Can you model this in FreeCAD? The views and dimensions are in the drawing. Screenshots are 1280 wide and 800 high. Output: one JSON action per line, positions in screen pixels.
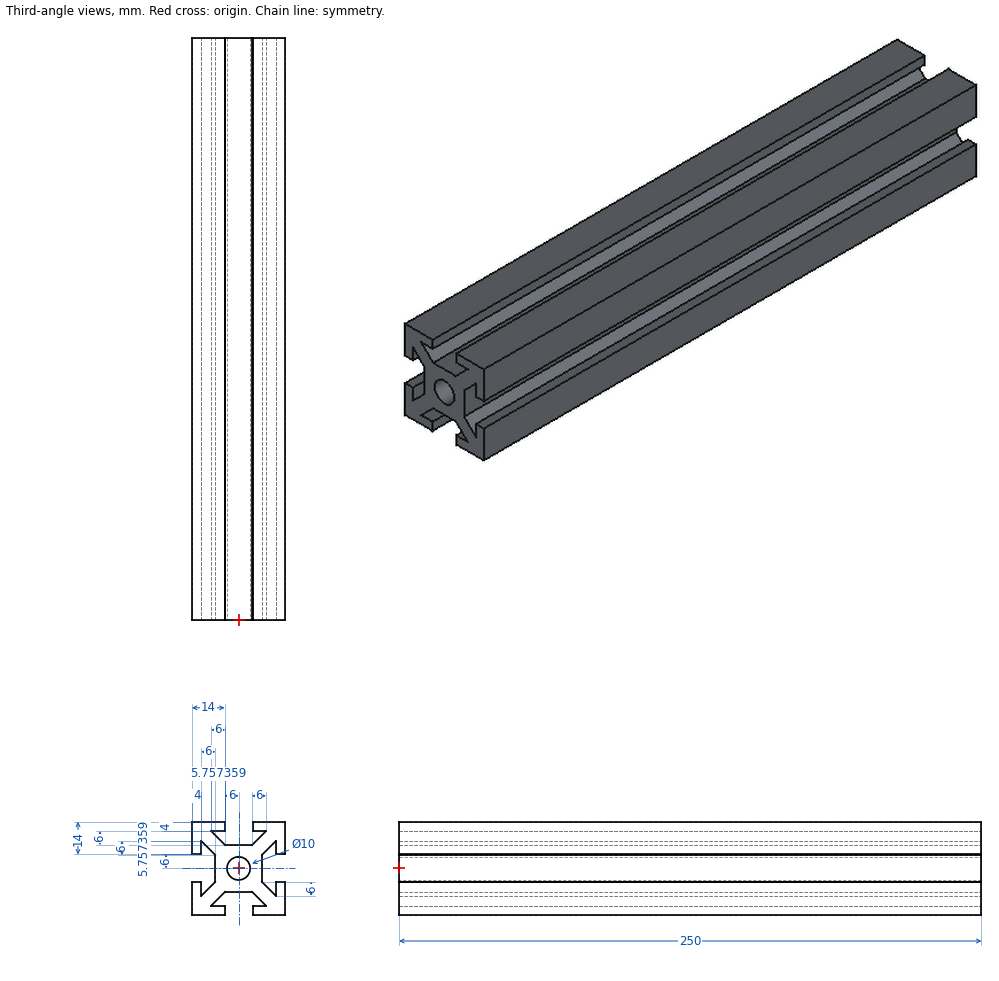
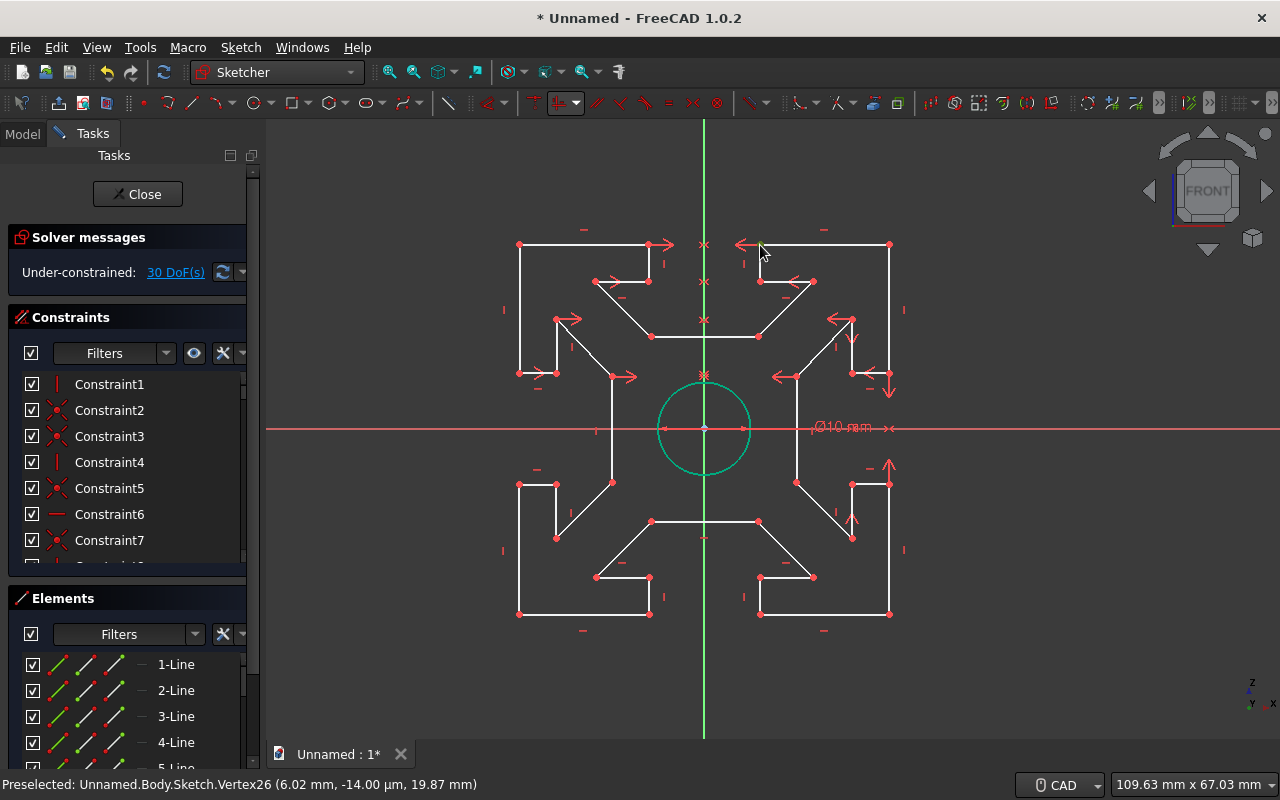
{"action": "left_click", "coordinate": [760, 615]}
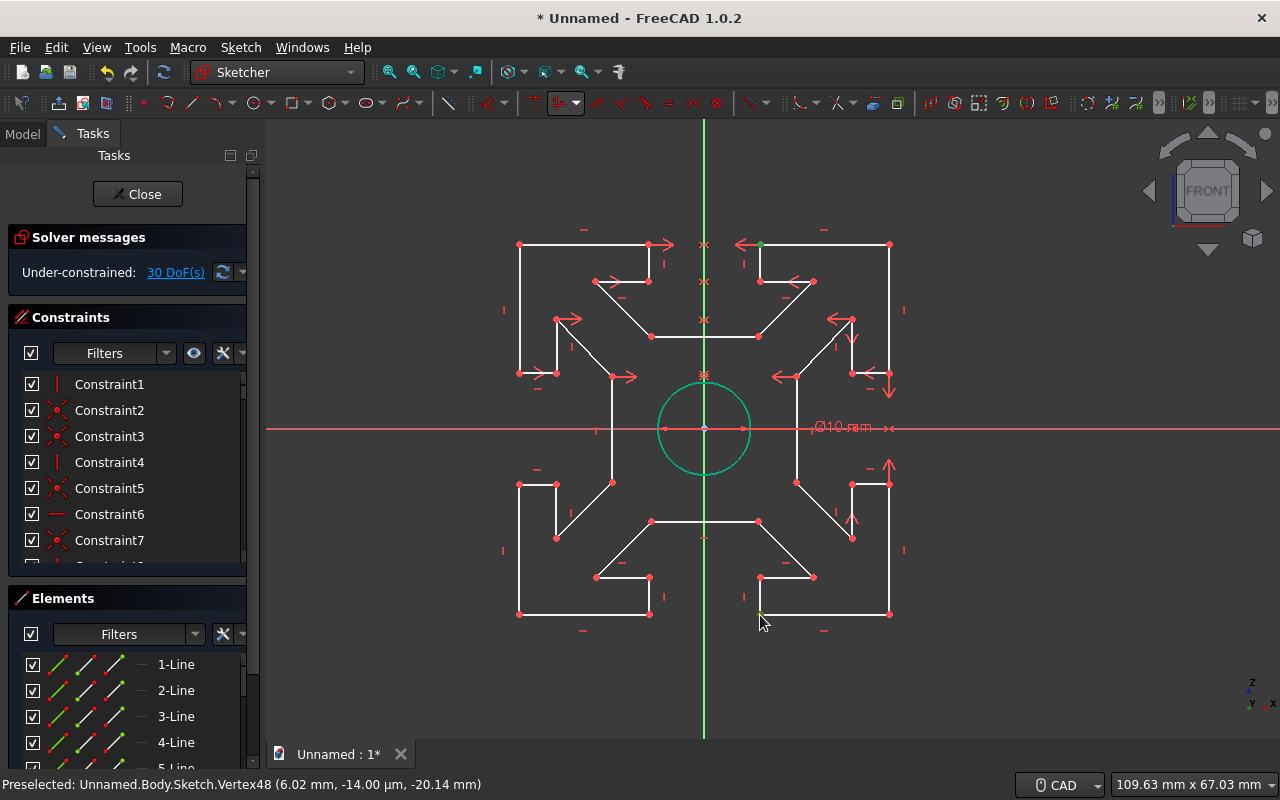
{"action": "left_click", "coordinate": [353, 429]}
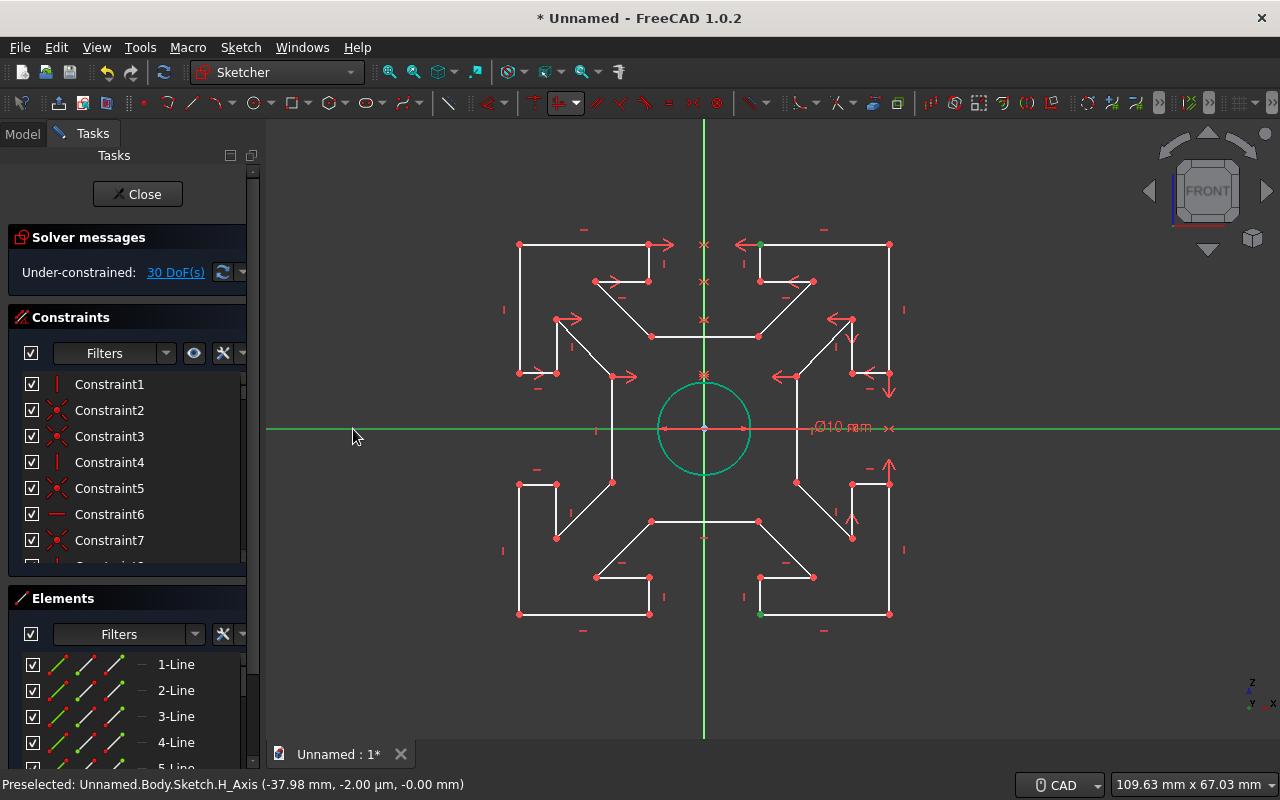
{"action": "left_click", "coordinate": [694, 104]}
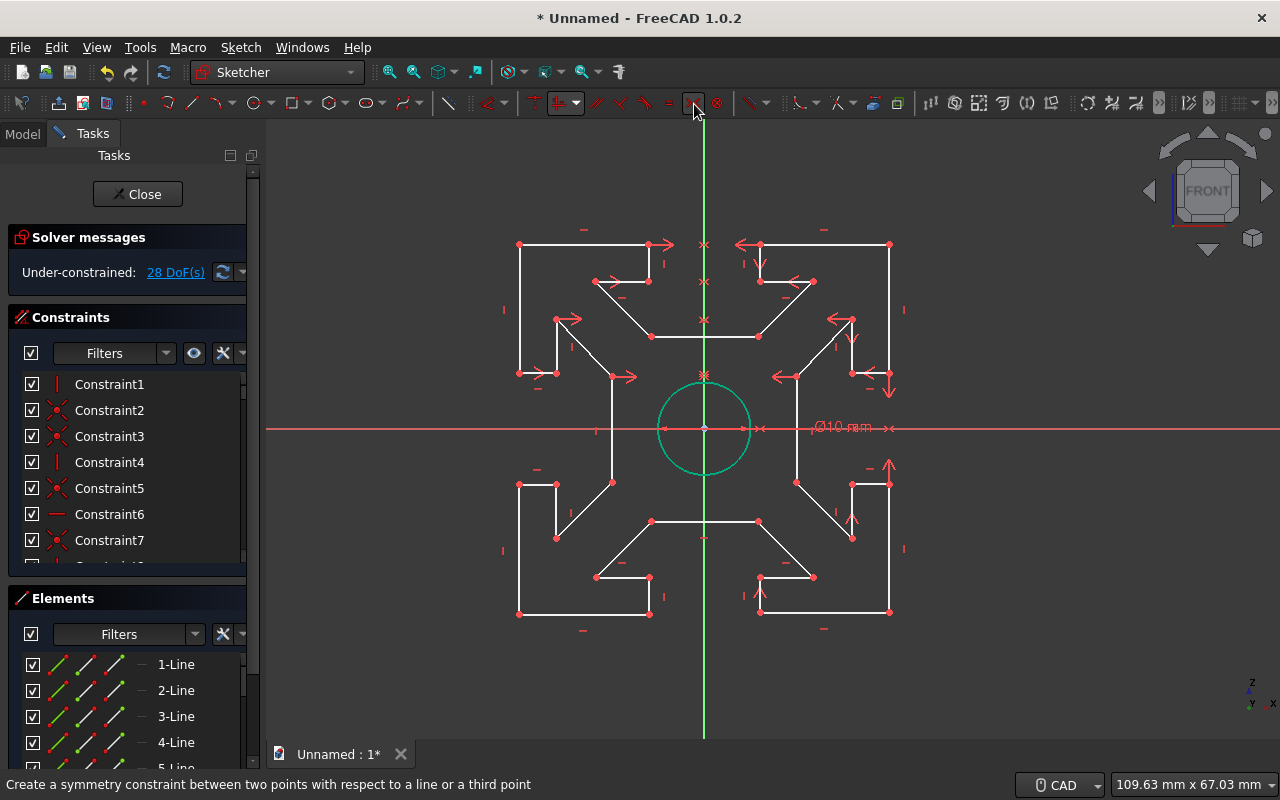
{"action": "left_click", "coordinate": [813, 282]}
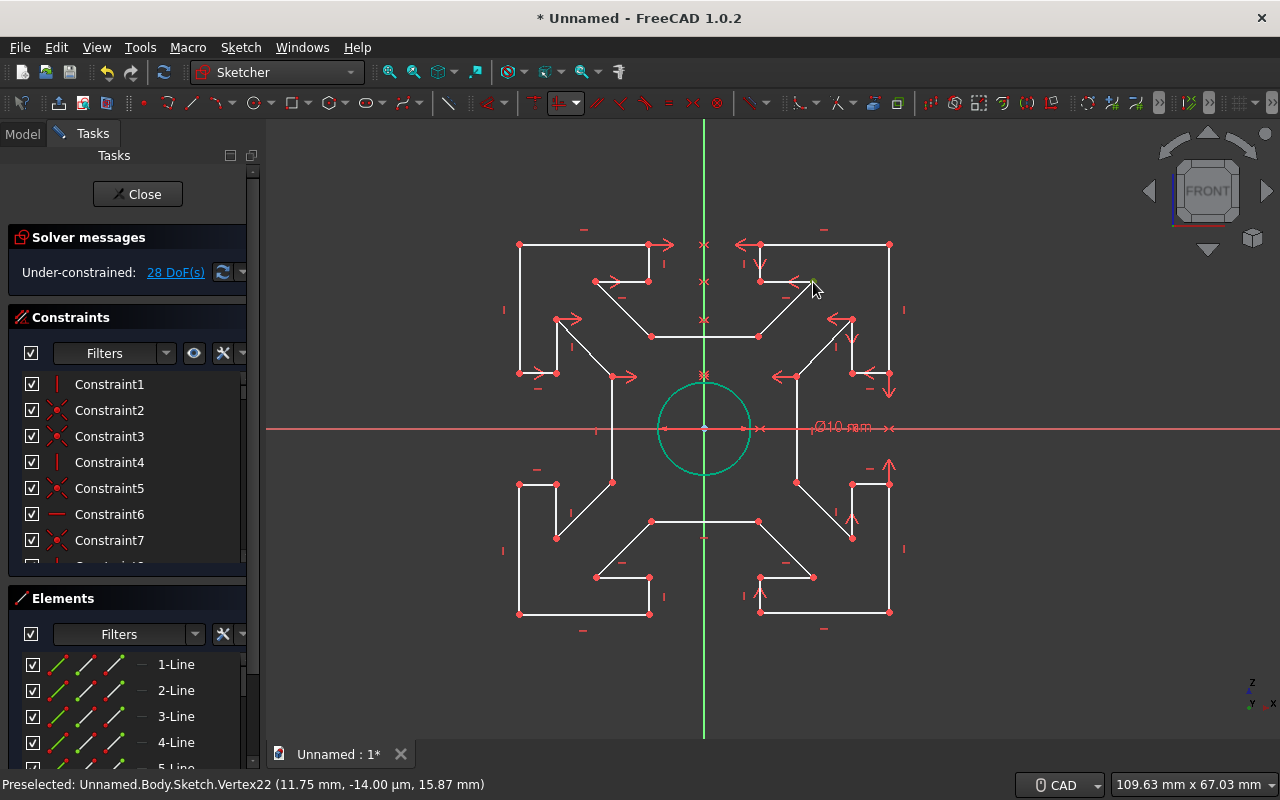
{"action": "left_click", "coordinate": [813, 578]}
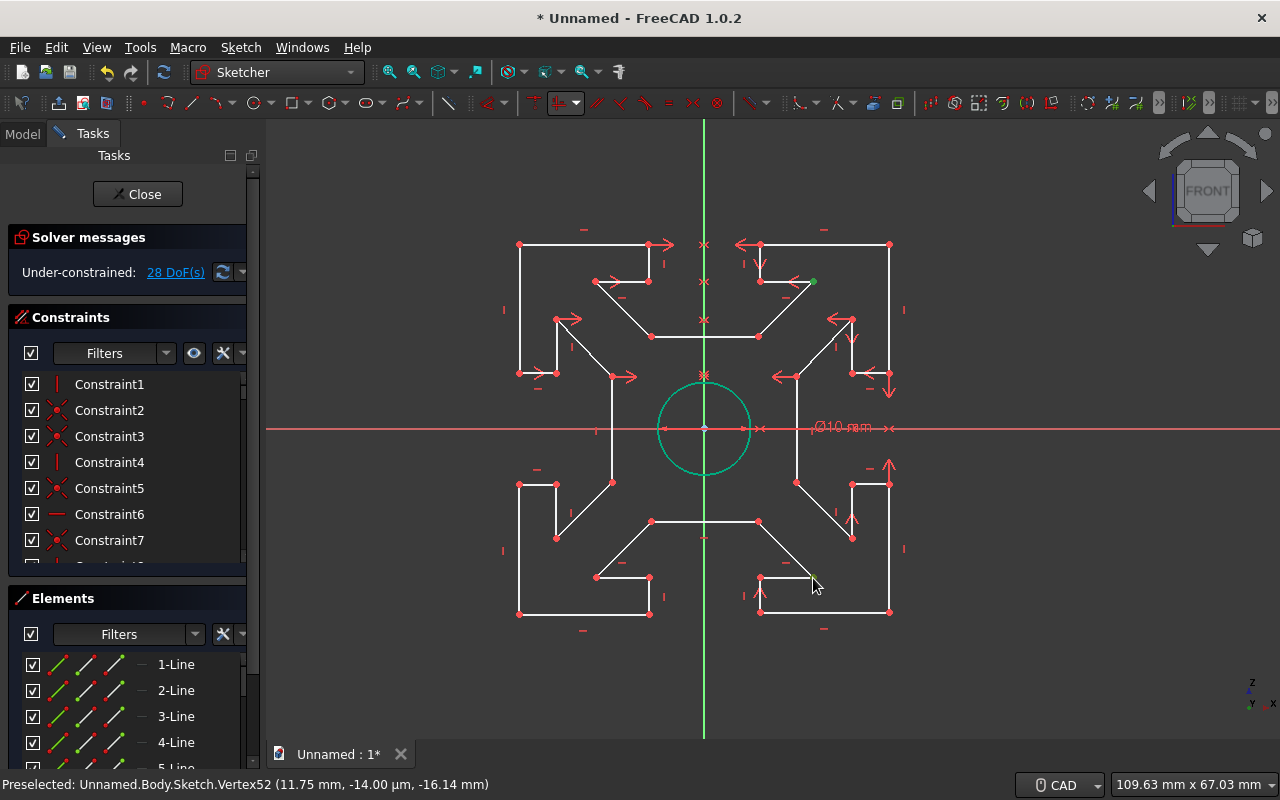
{"action": "left_click", "coordinate": [353, 429]}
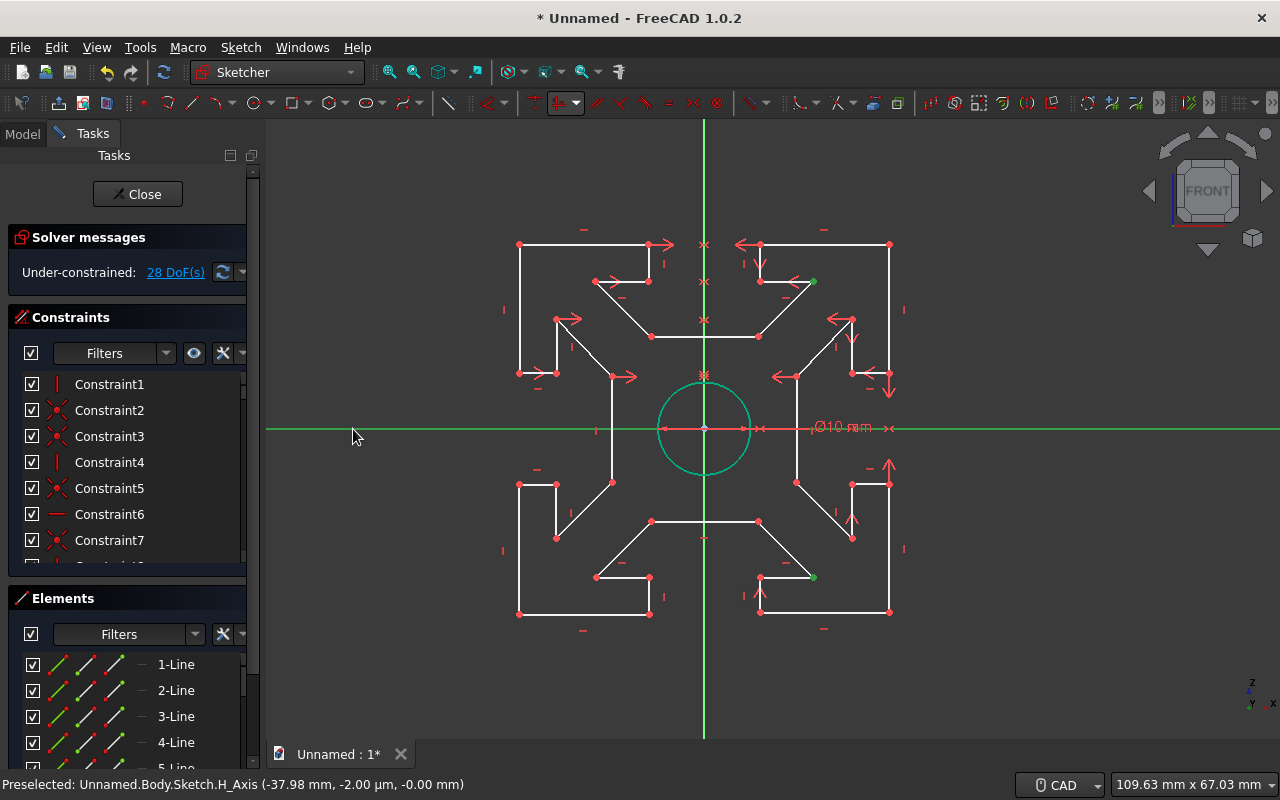
{"action": "left_click", "coordinate": [694, 104]}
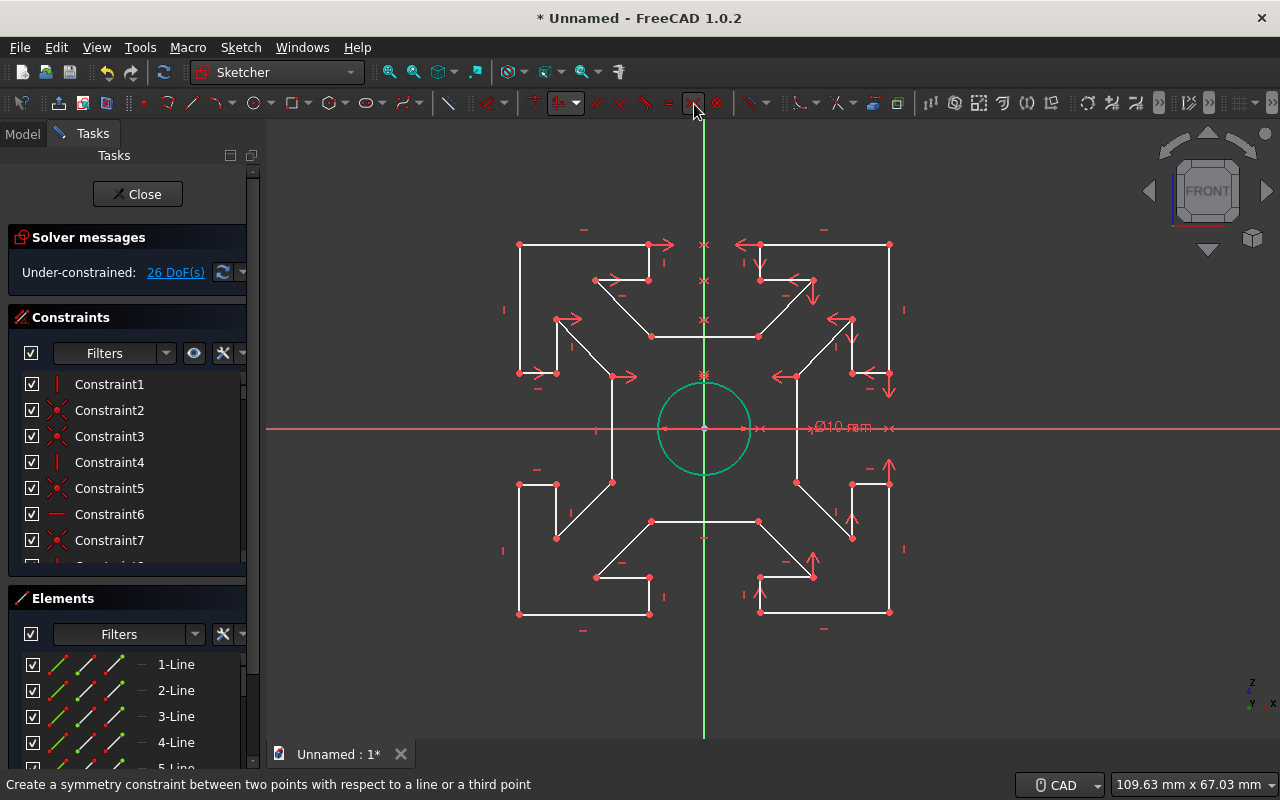
{"action": "left_click", "coordinate": [758, 337]}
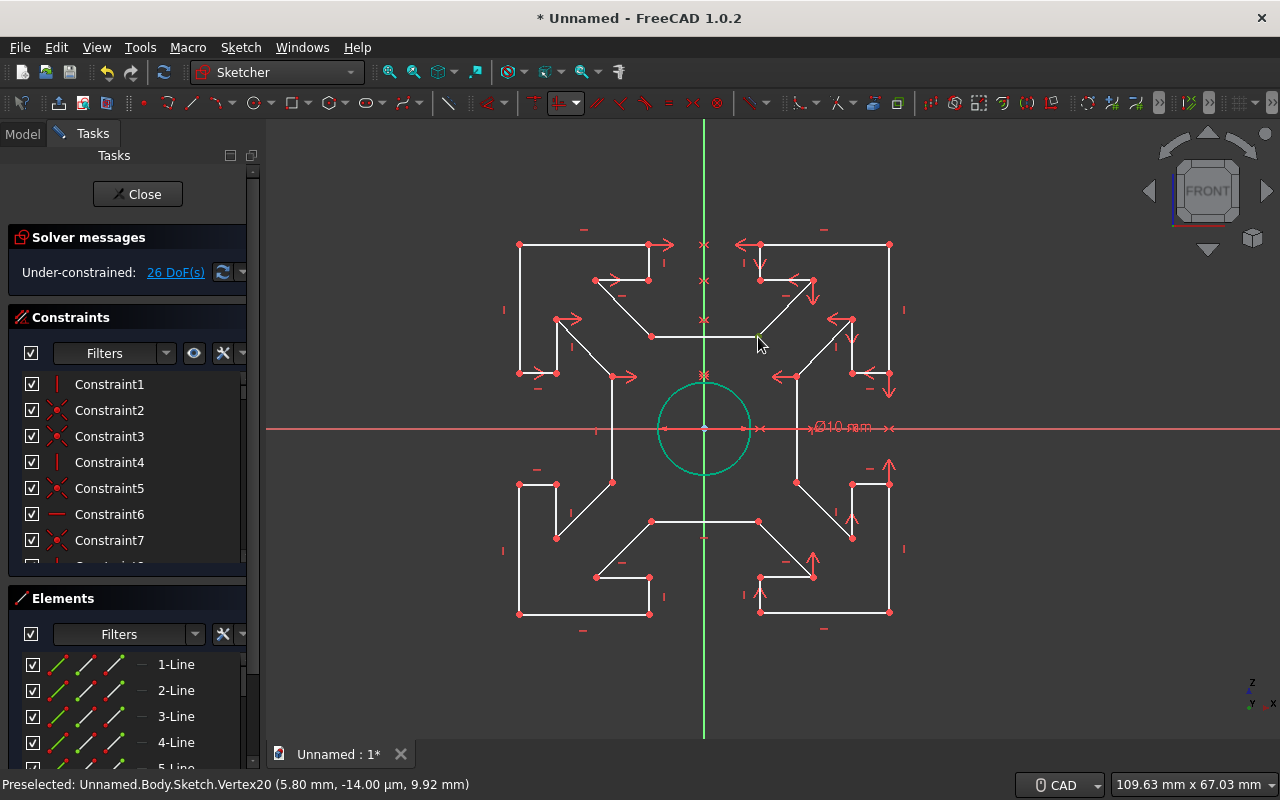
{"action": "left_click", "coordinate": [758, 522]}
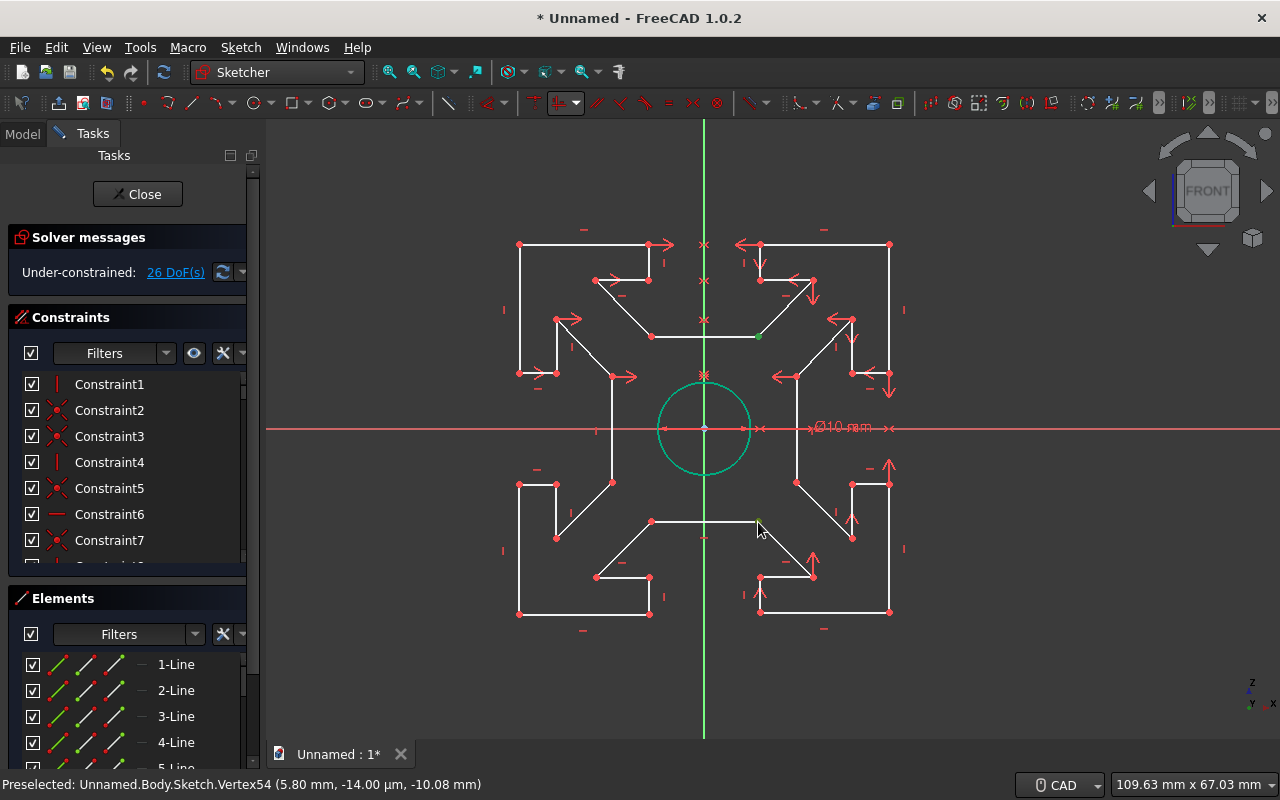
{"action": "left_click", "coordinate": [353, 429]}